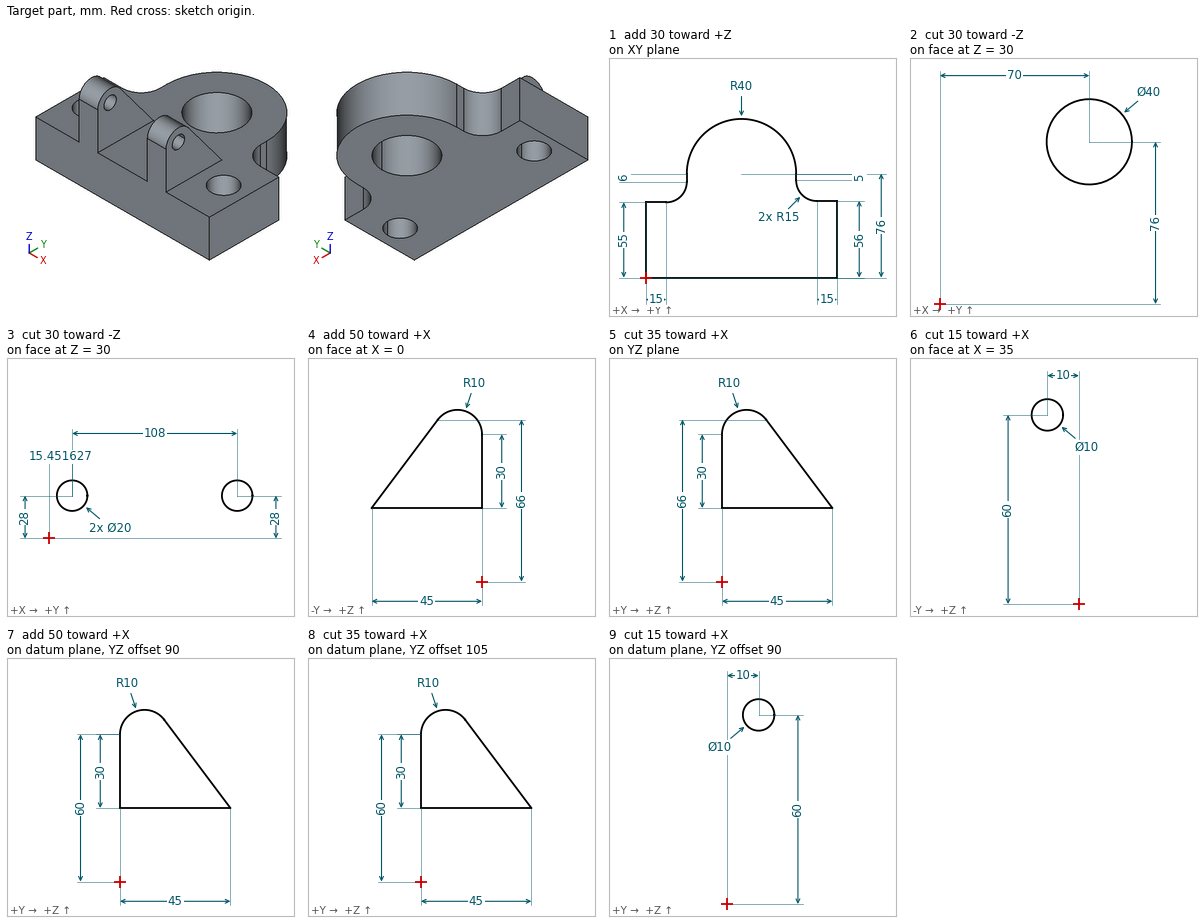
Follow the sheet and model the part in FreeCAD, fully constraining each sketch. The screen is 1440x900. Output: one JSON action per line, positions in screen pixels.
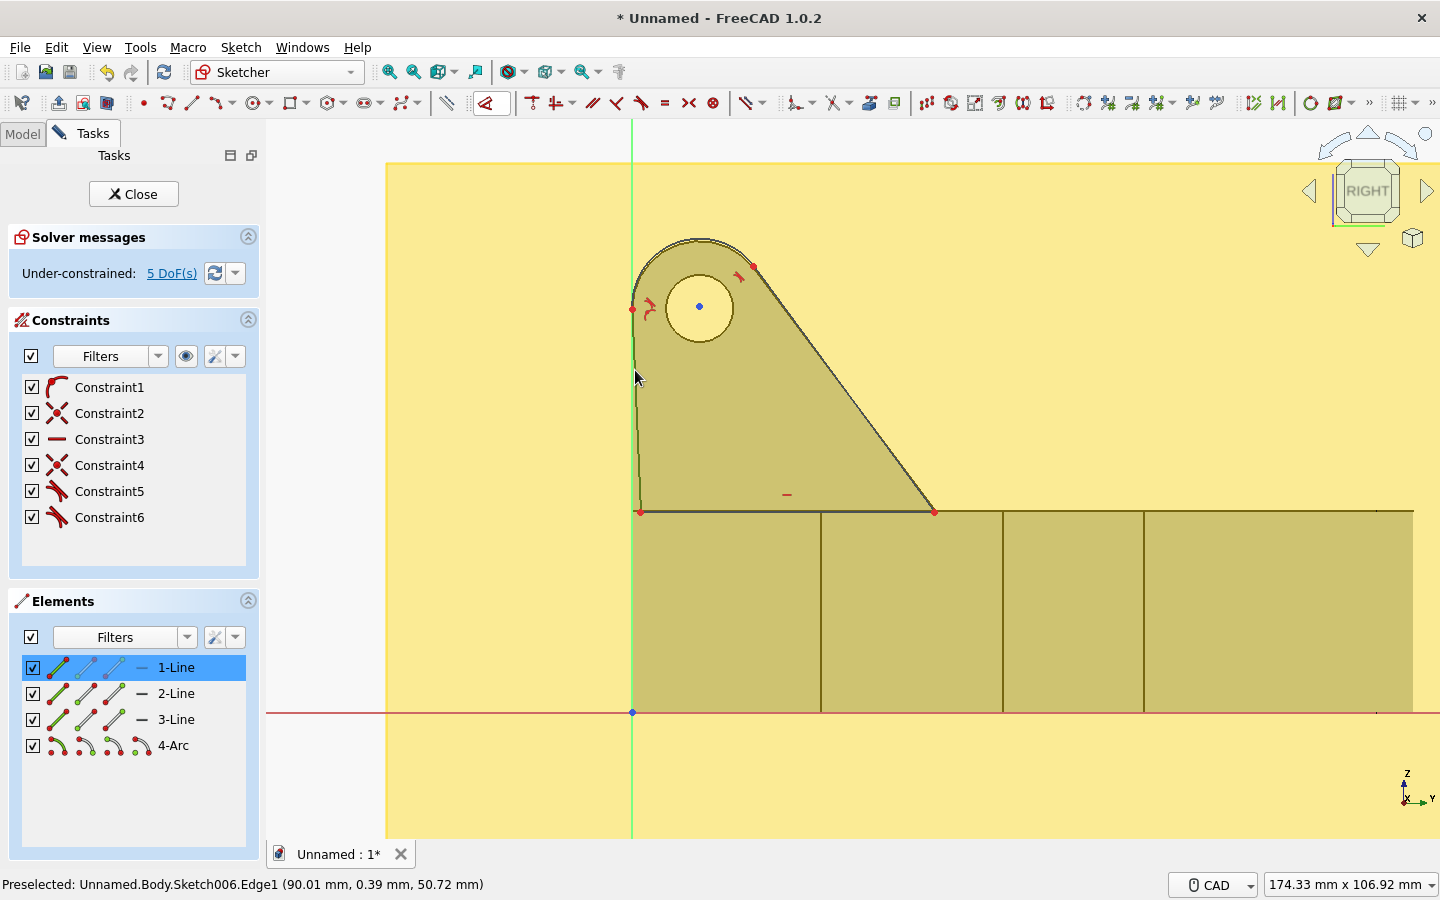
{"action": "key", "text": "v"}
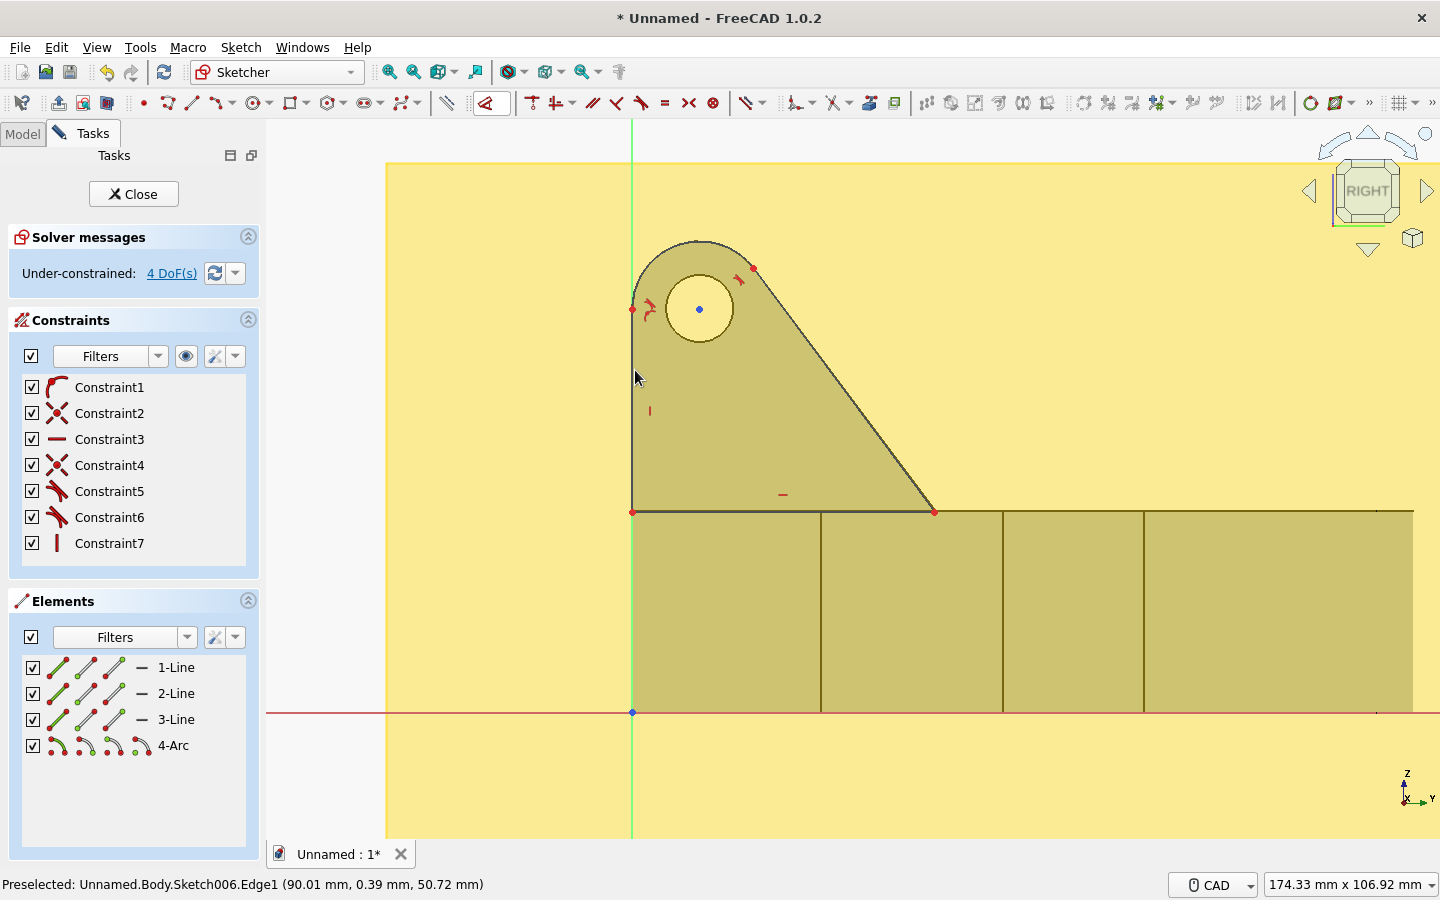
{"action": "left_click", "coordinate": [712, 243]}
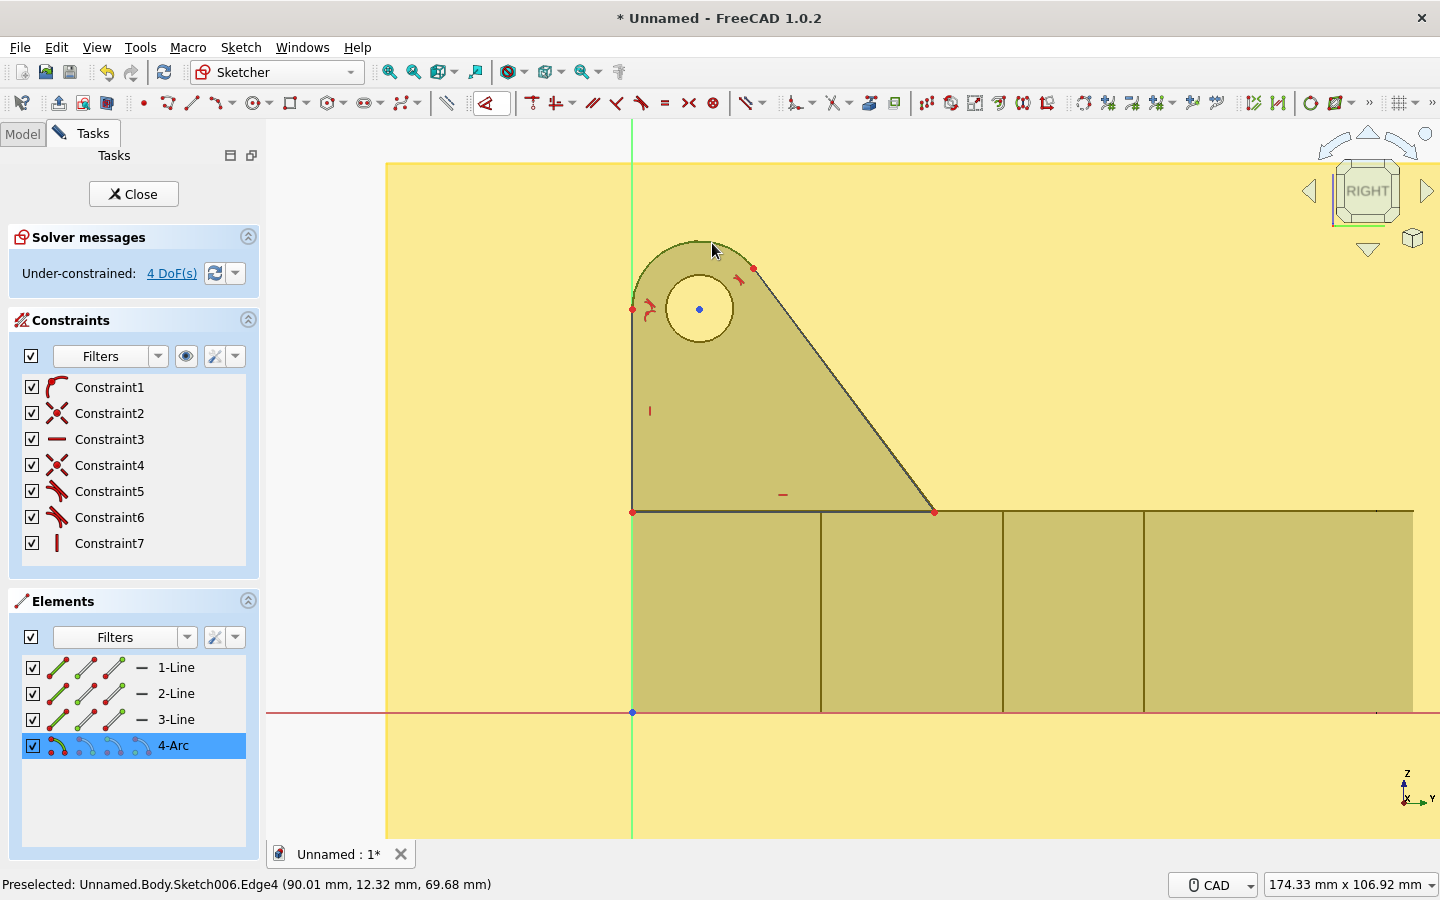
{"action": "key", "text": "k r"}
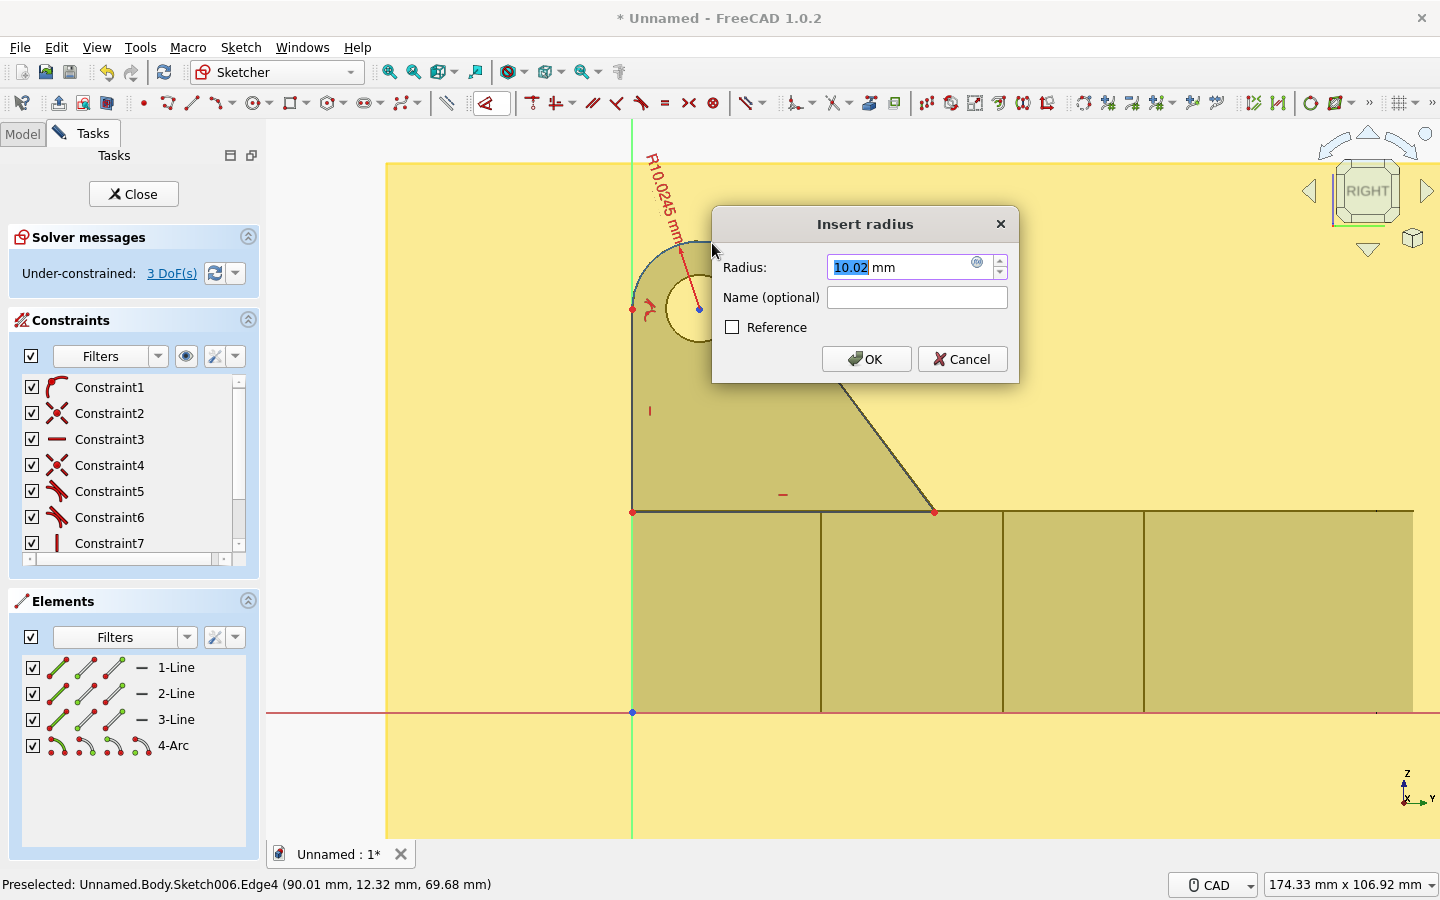
{"action": "type", "text": "10"}
{"action": "key", "text": "Return"}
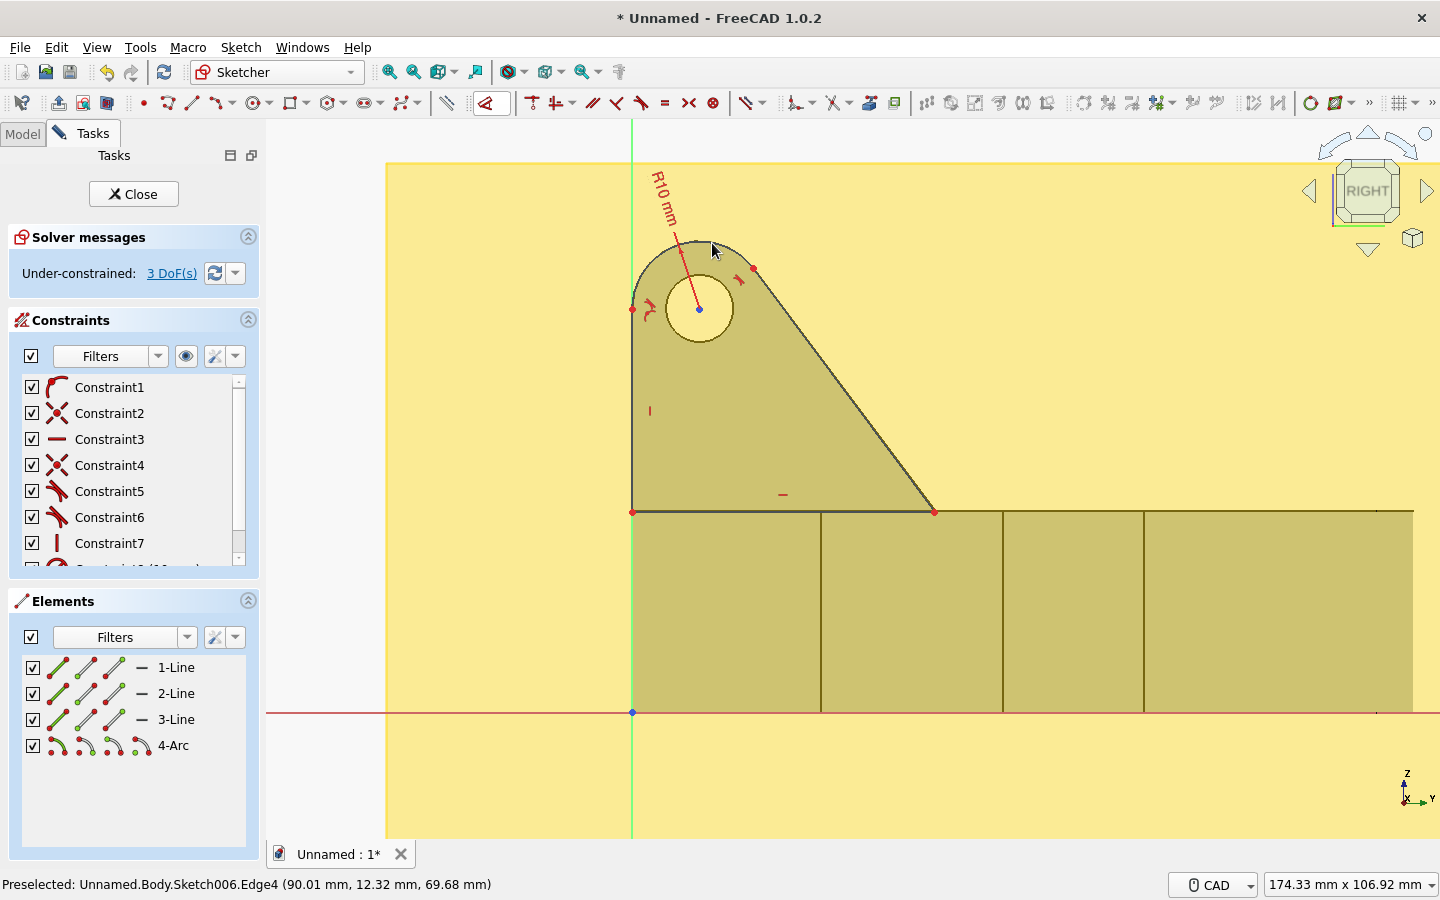
{"action": "left_click", "coordinate": [632, 370]}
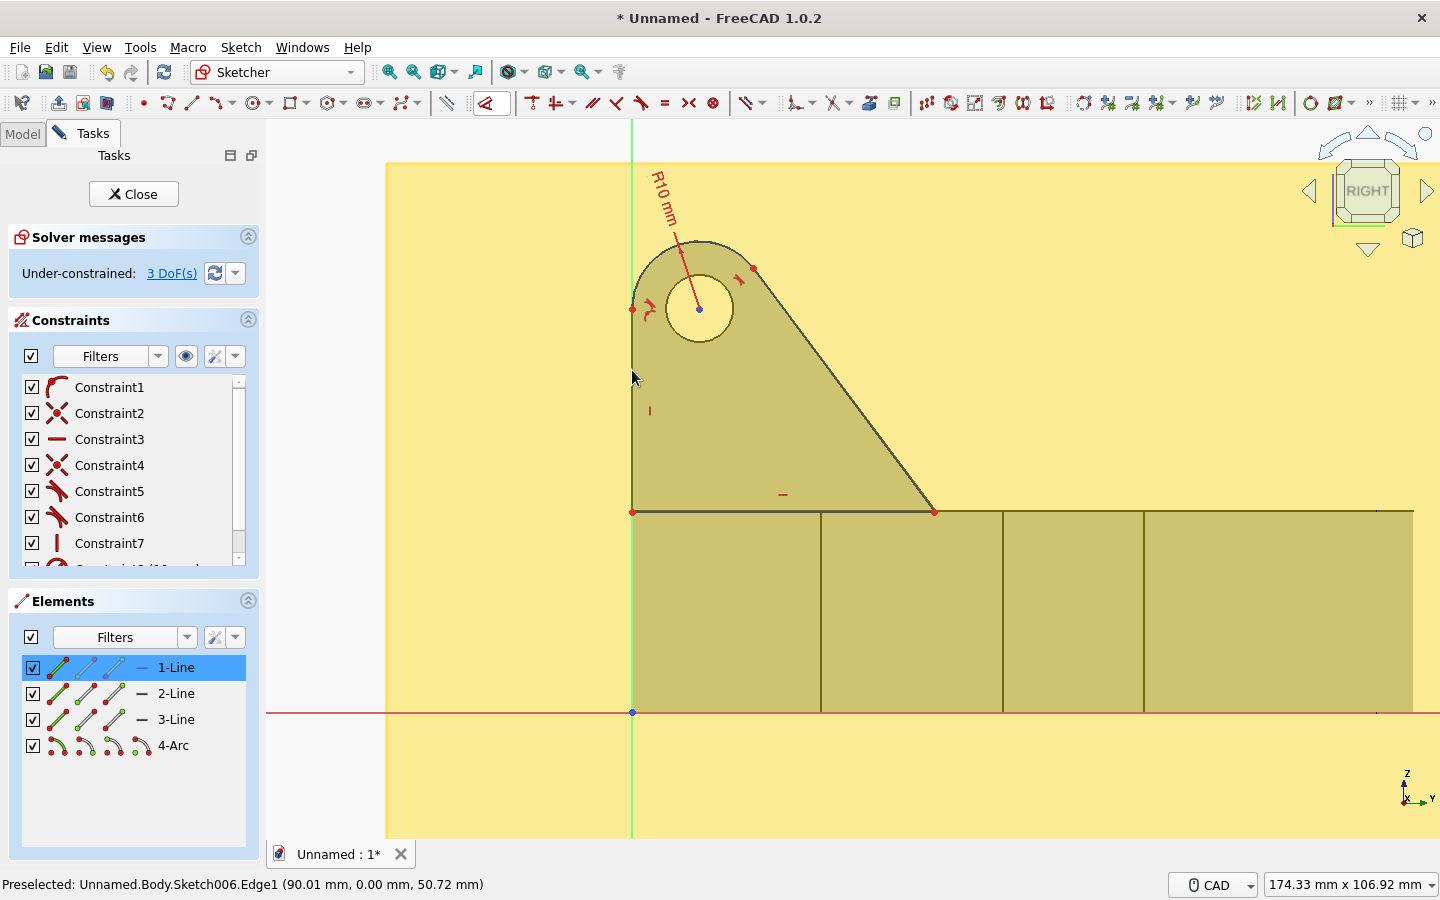
{"action": "key", "text": "i"}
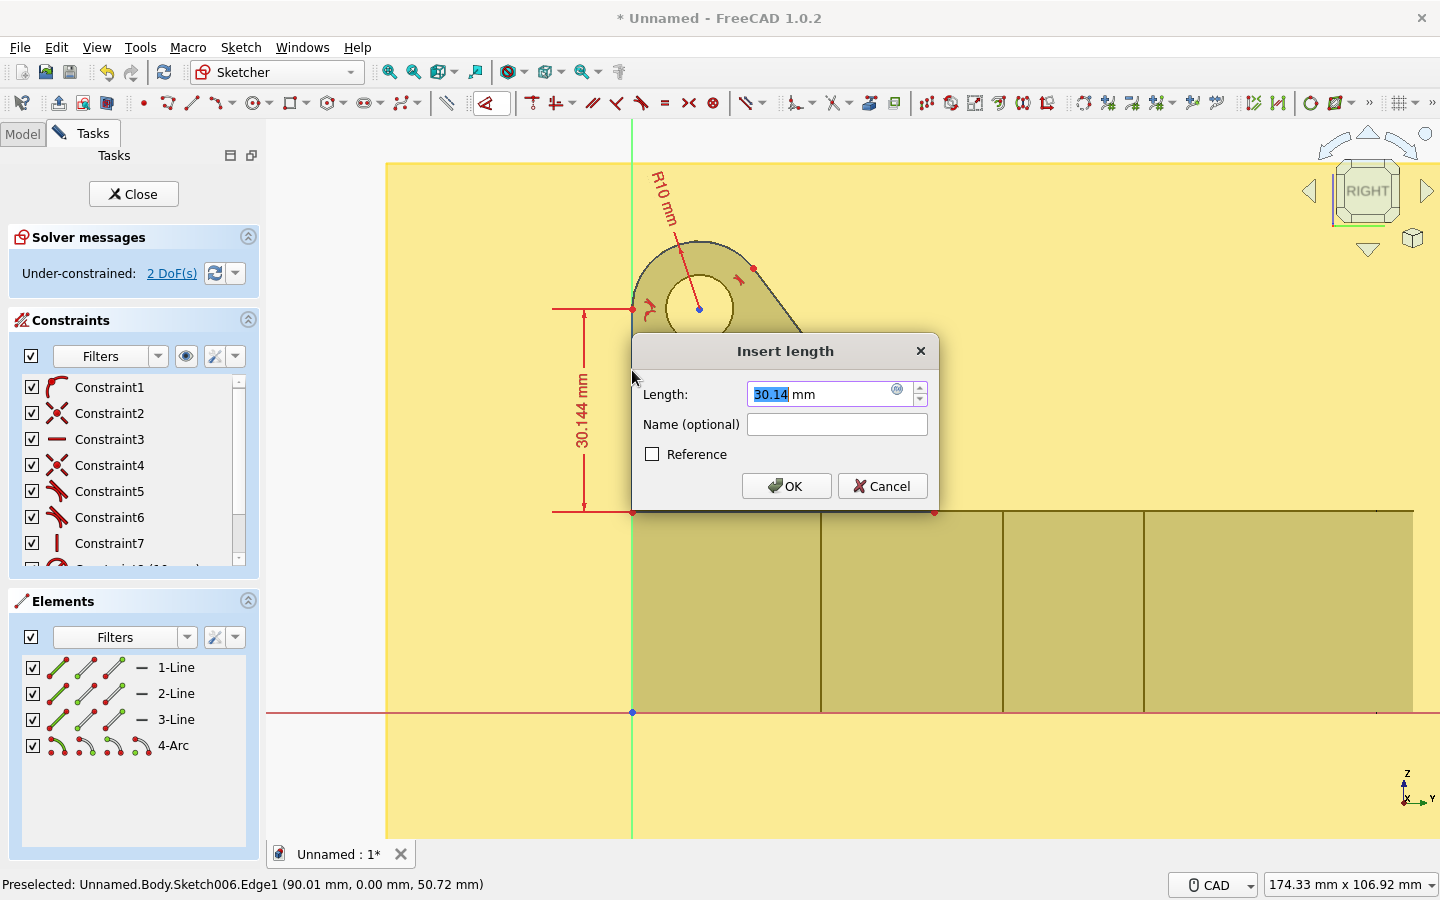
{"action": "type", "text": "30"}
{"action": "key", "text": "Return"}